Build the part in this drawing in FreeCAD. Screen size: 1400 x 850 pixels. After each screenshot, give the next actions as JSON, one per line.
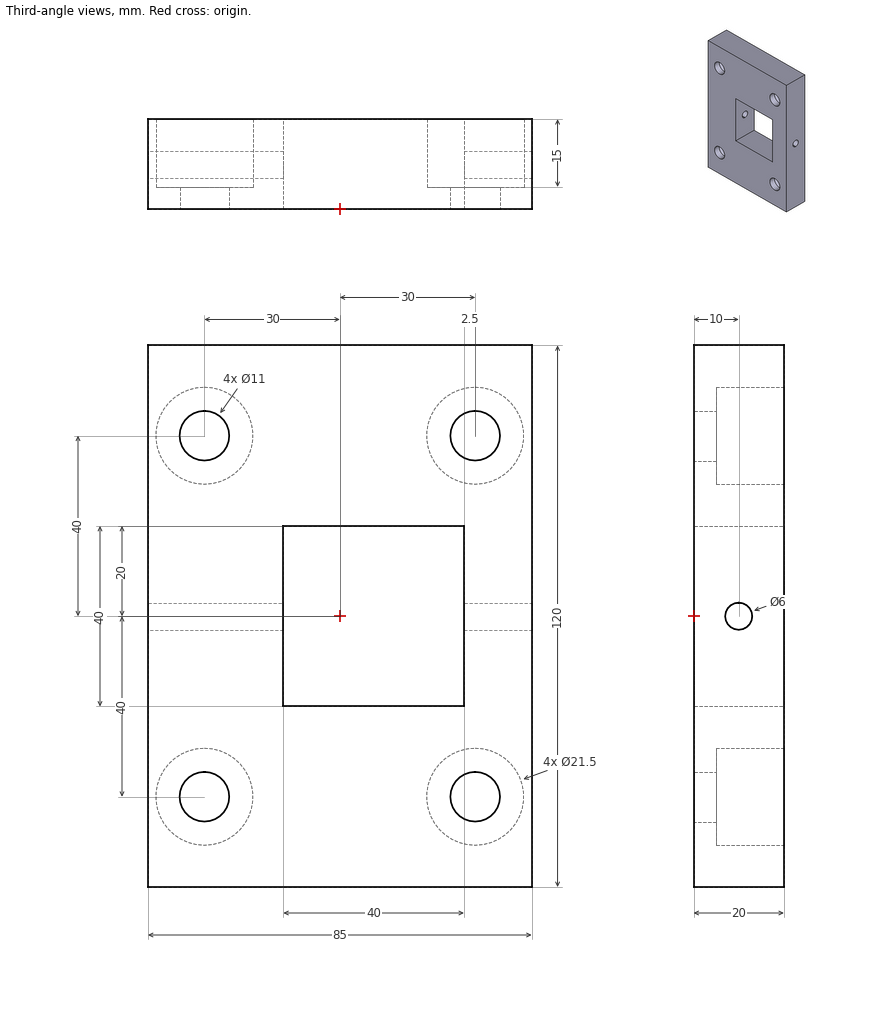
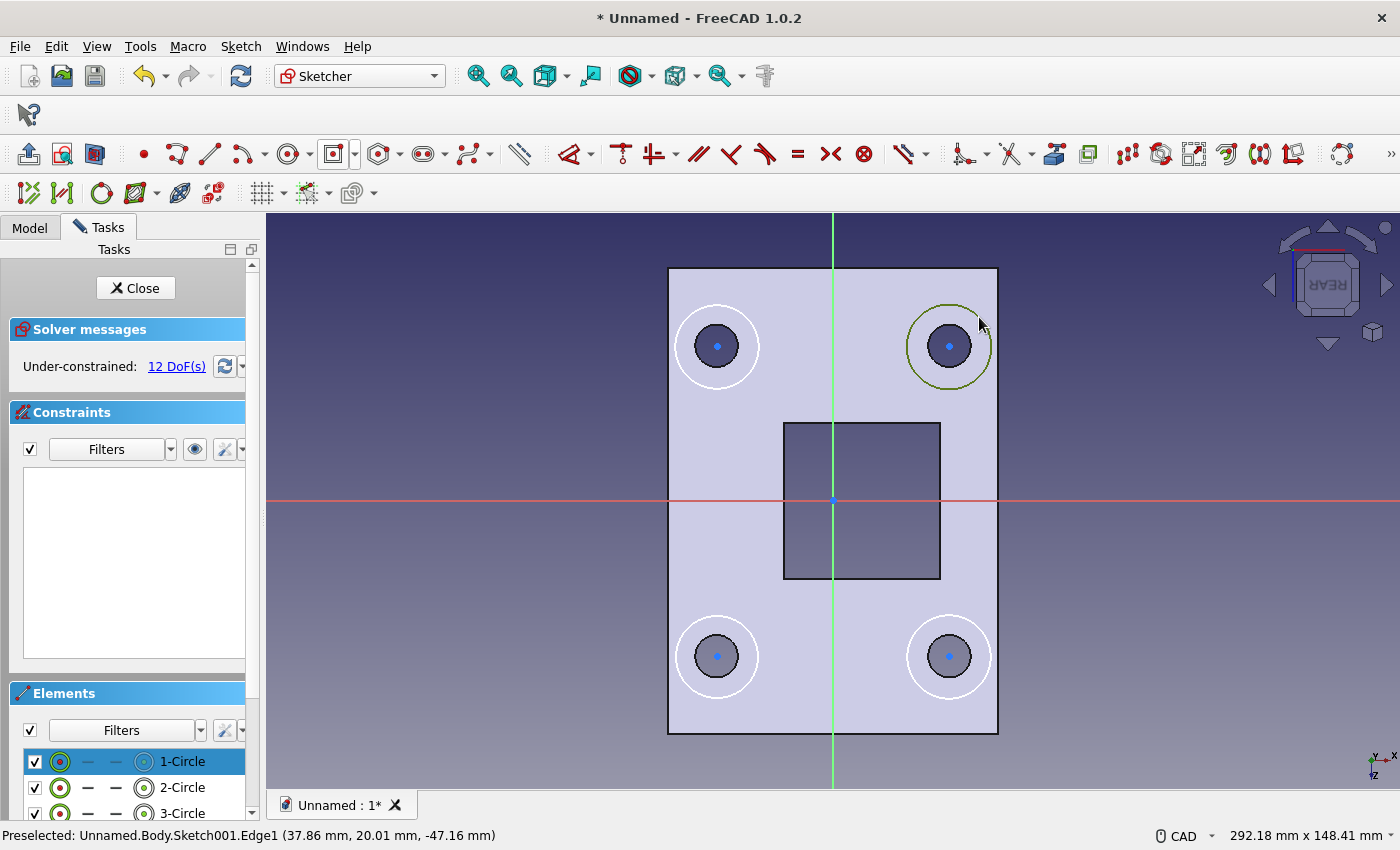
{"action": "left_click", "coordinate": [746, 317]}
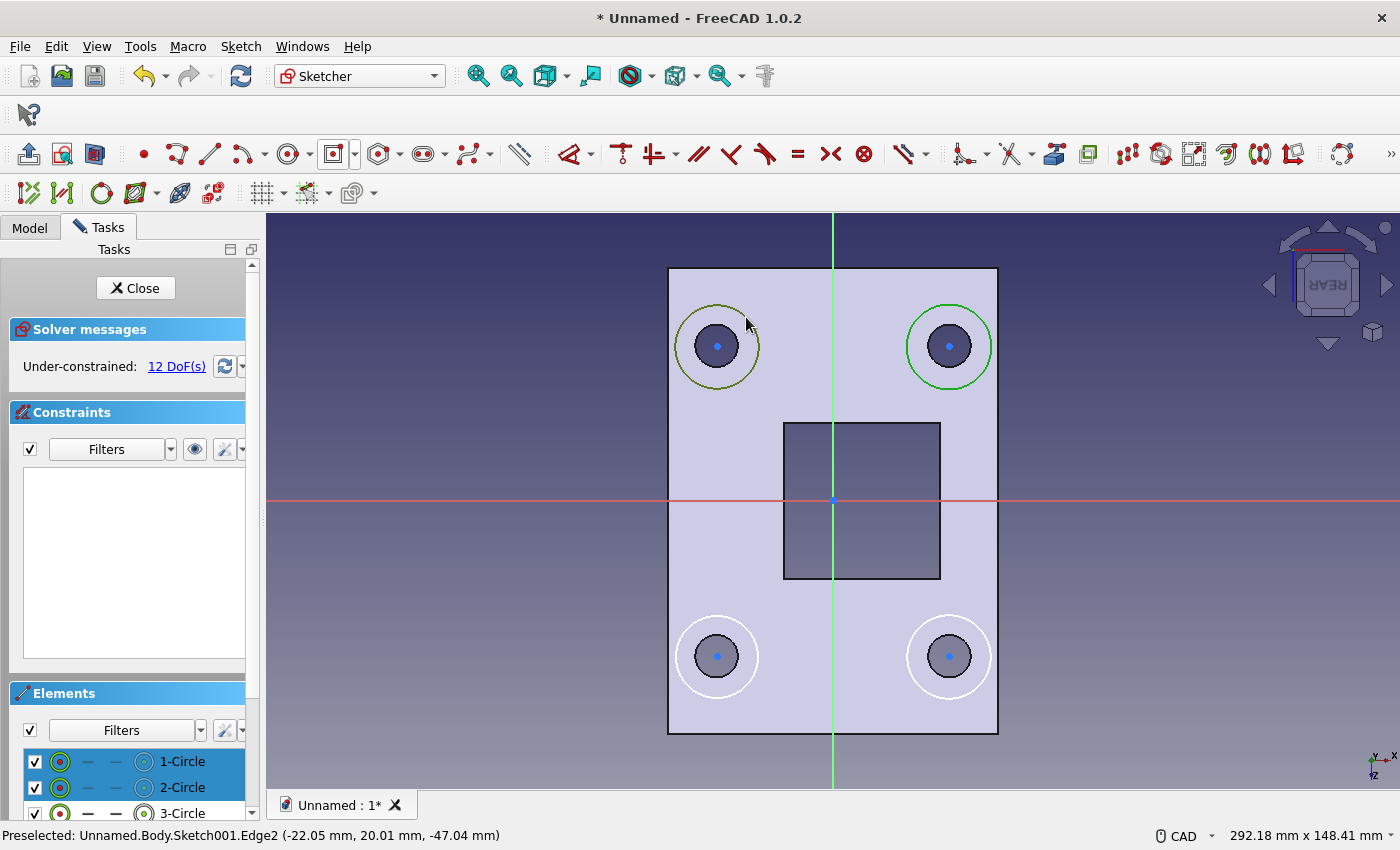
{"action": "left_click", "coordinate": [746, 628]}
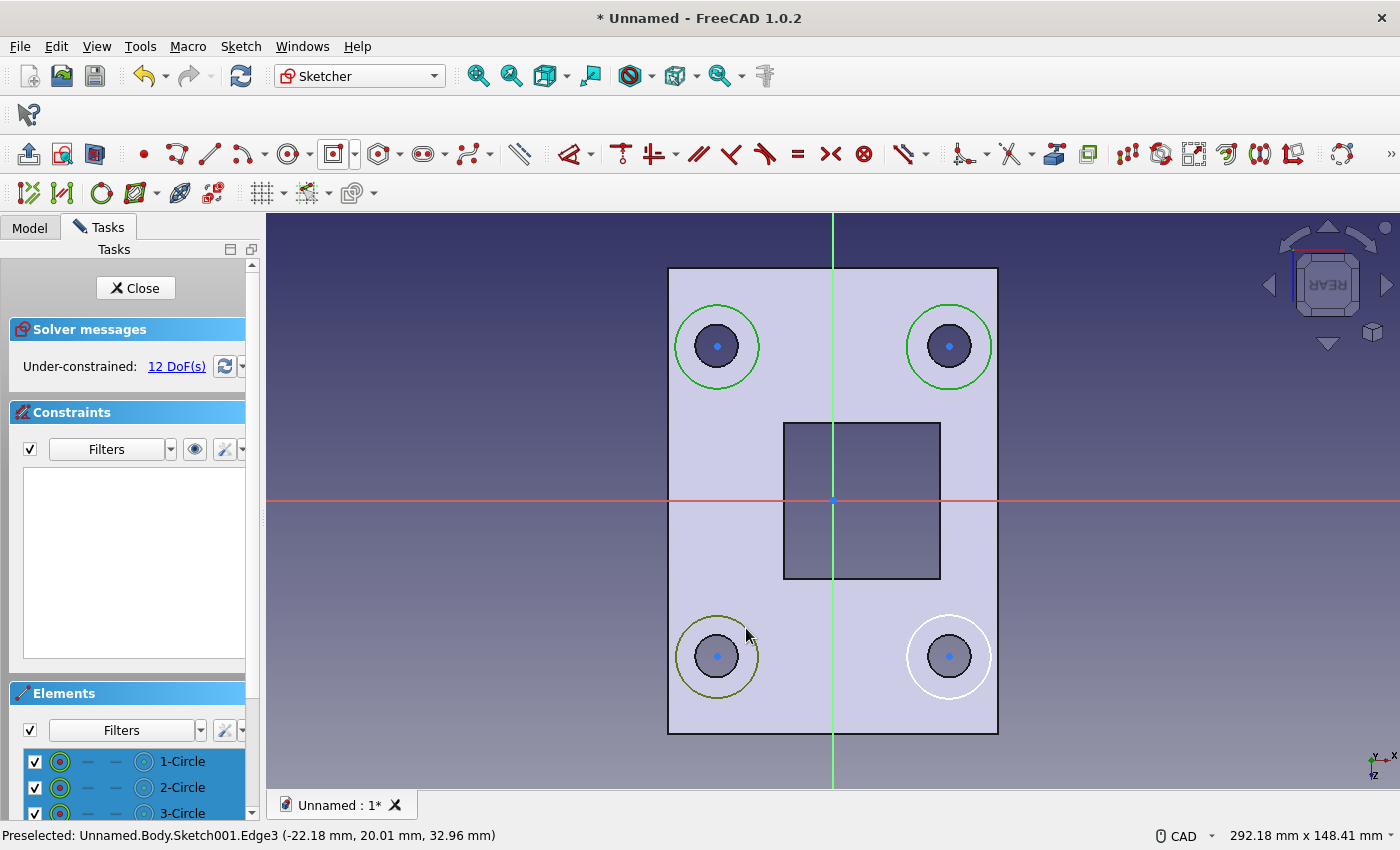
{"action": "left_click", "coordinate": [978, 627]}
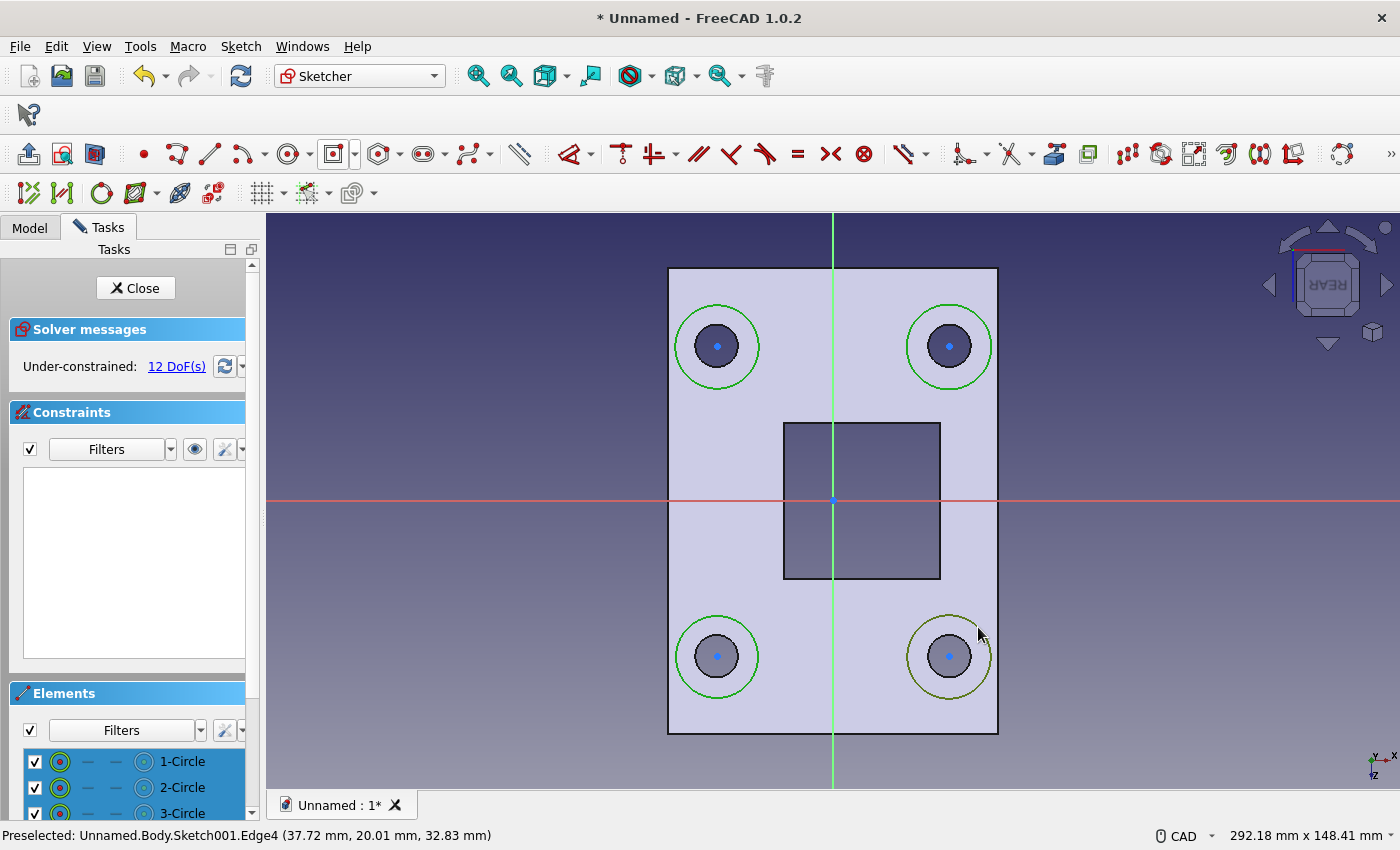
{"action": "left_click", "coordinate": [798, 154]}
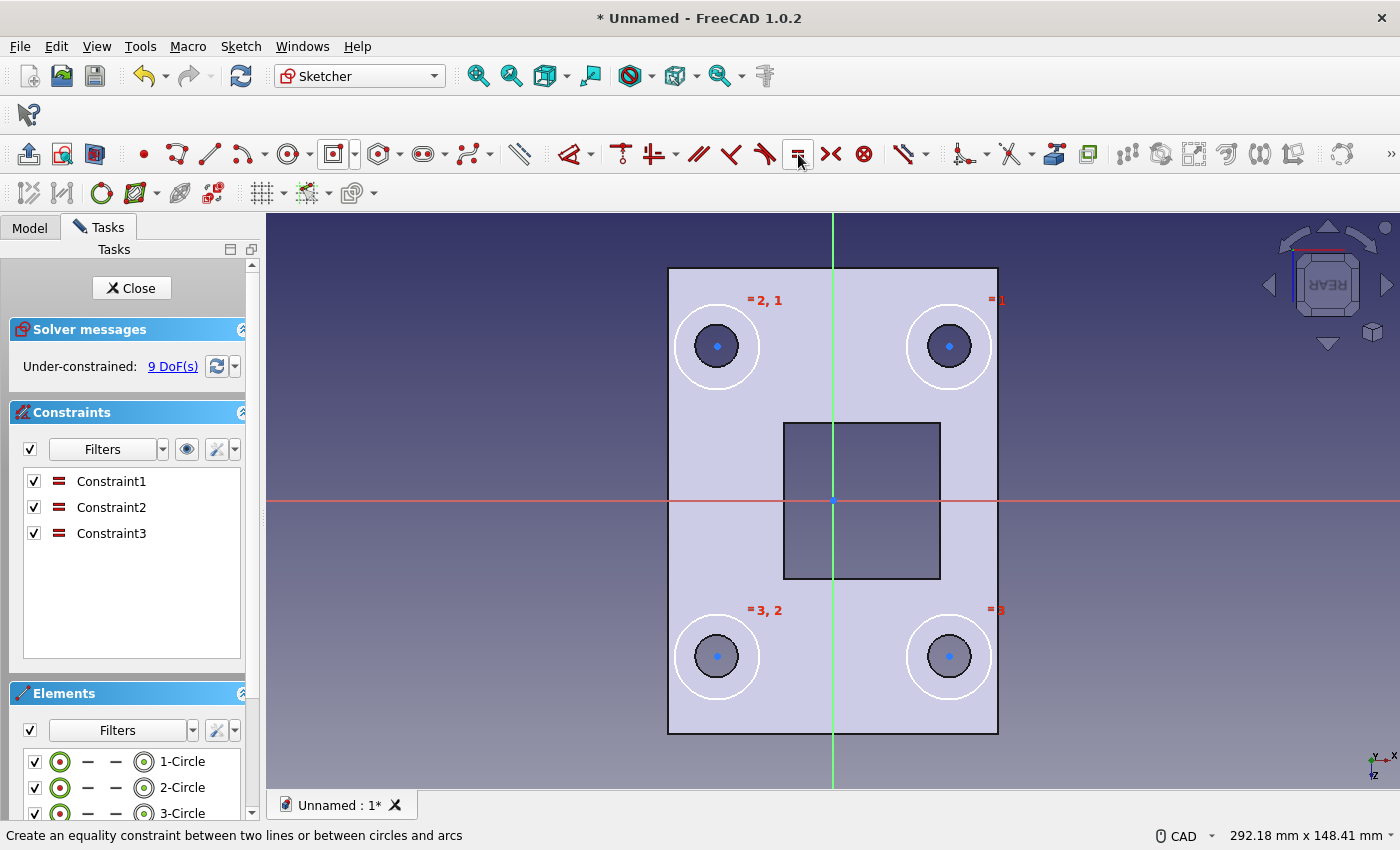
{"action": "key", "text": "d"}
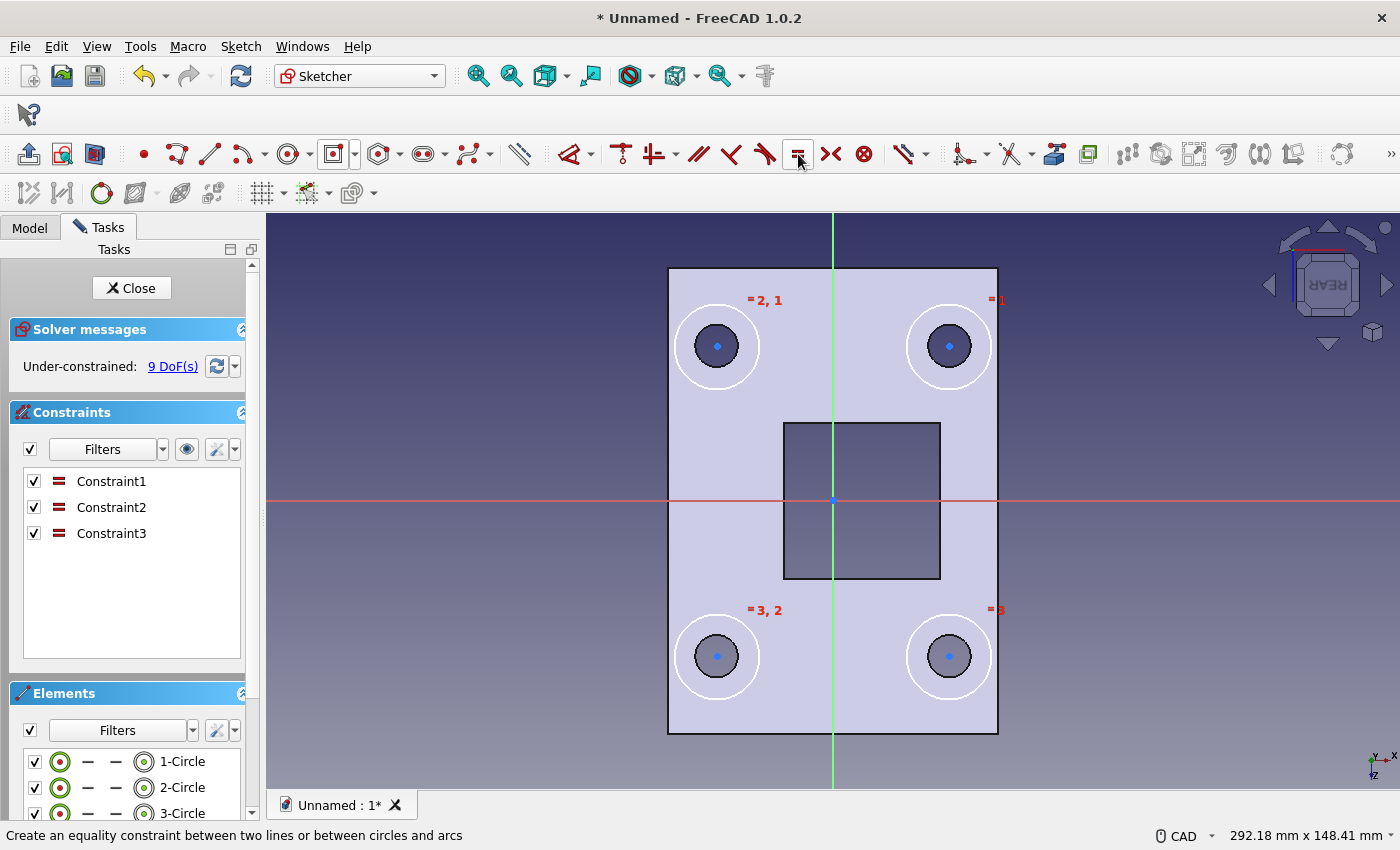
{"action": "left_click", "coordinate": [979, 317]}
{"action": "left_click", "coordinate": [1002, 294]}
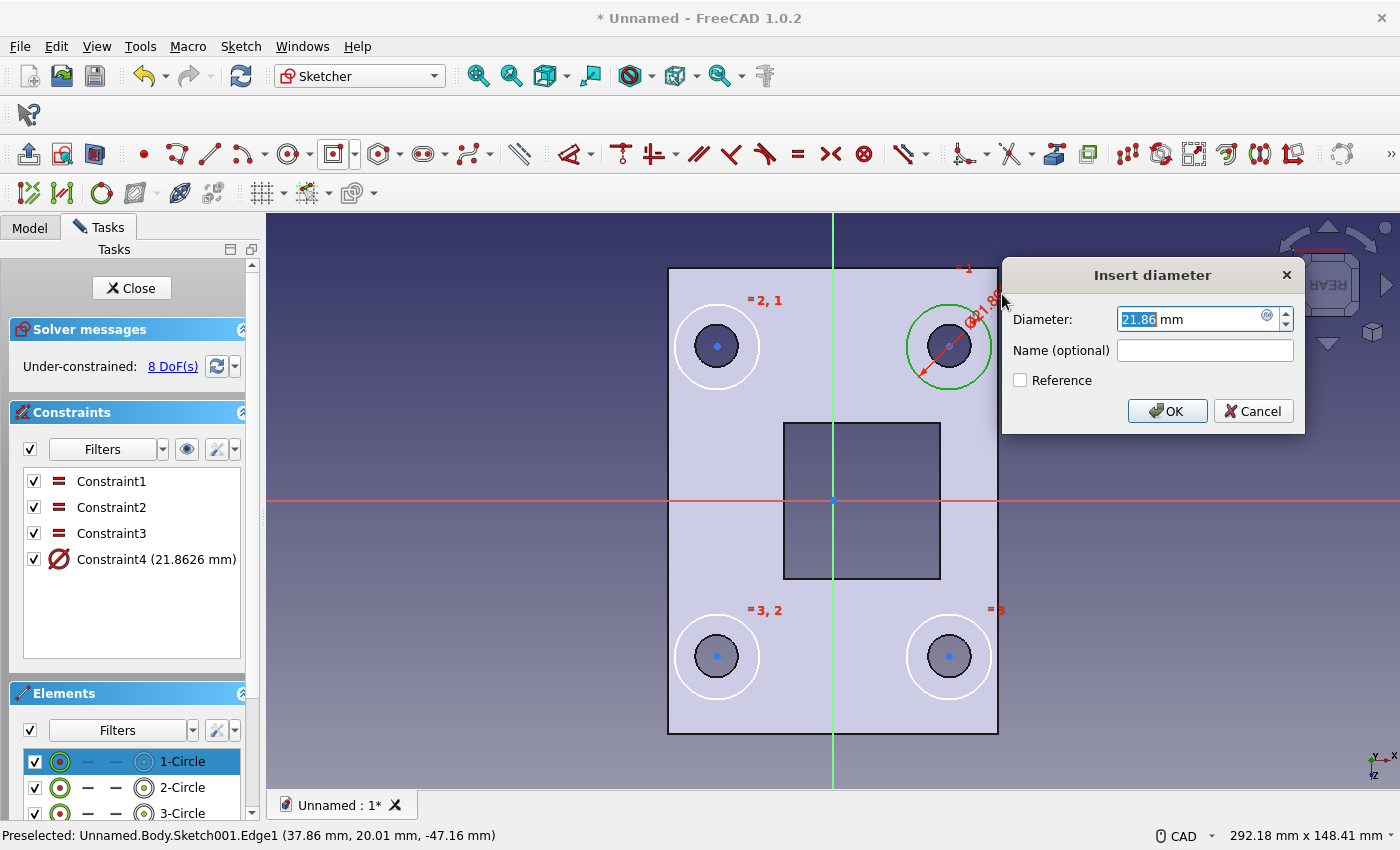
{"action": "type", "text": "21.5"}
{"action": "key", "text": "Return"}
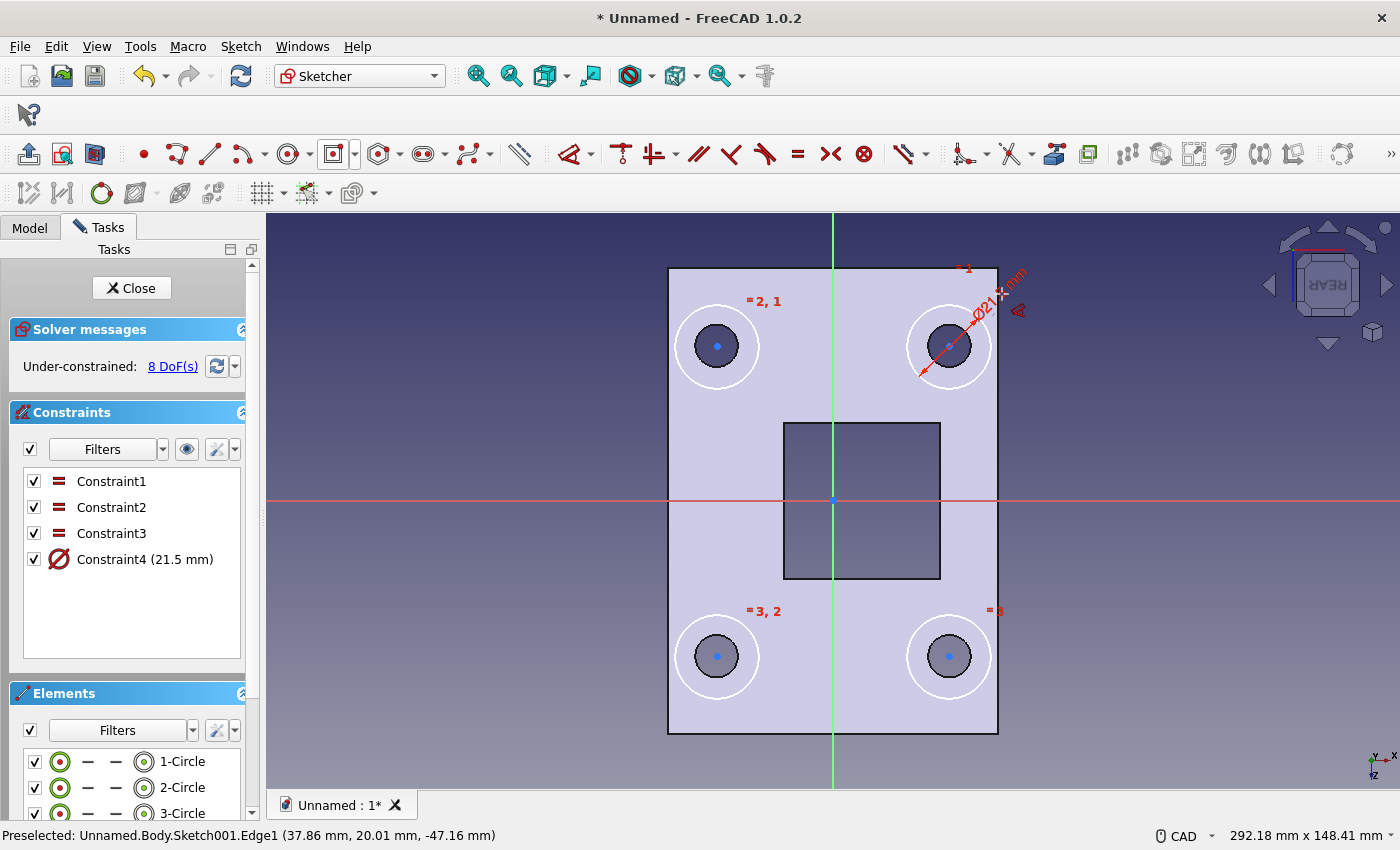
{"action": "left_click", "coordinate": [949, 347]}
{"action": "left_click", "coordinate": [891, 313]}